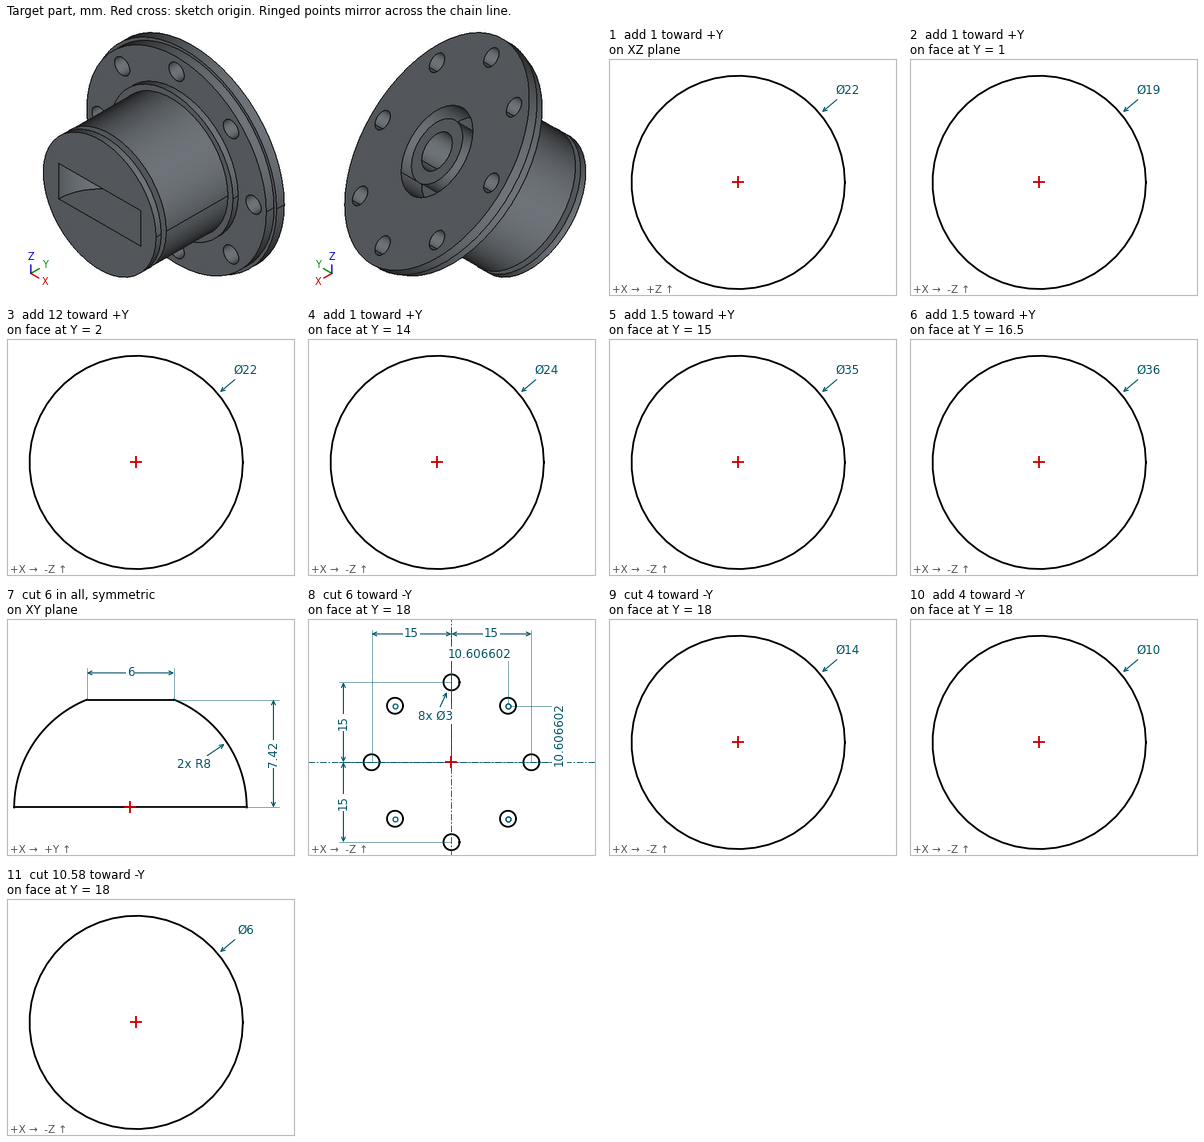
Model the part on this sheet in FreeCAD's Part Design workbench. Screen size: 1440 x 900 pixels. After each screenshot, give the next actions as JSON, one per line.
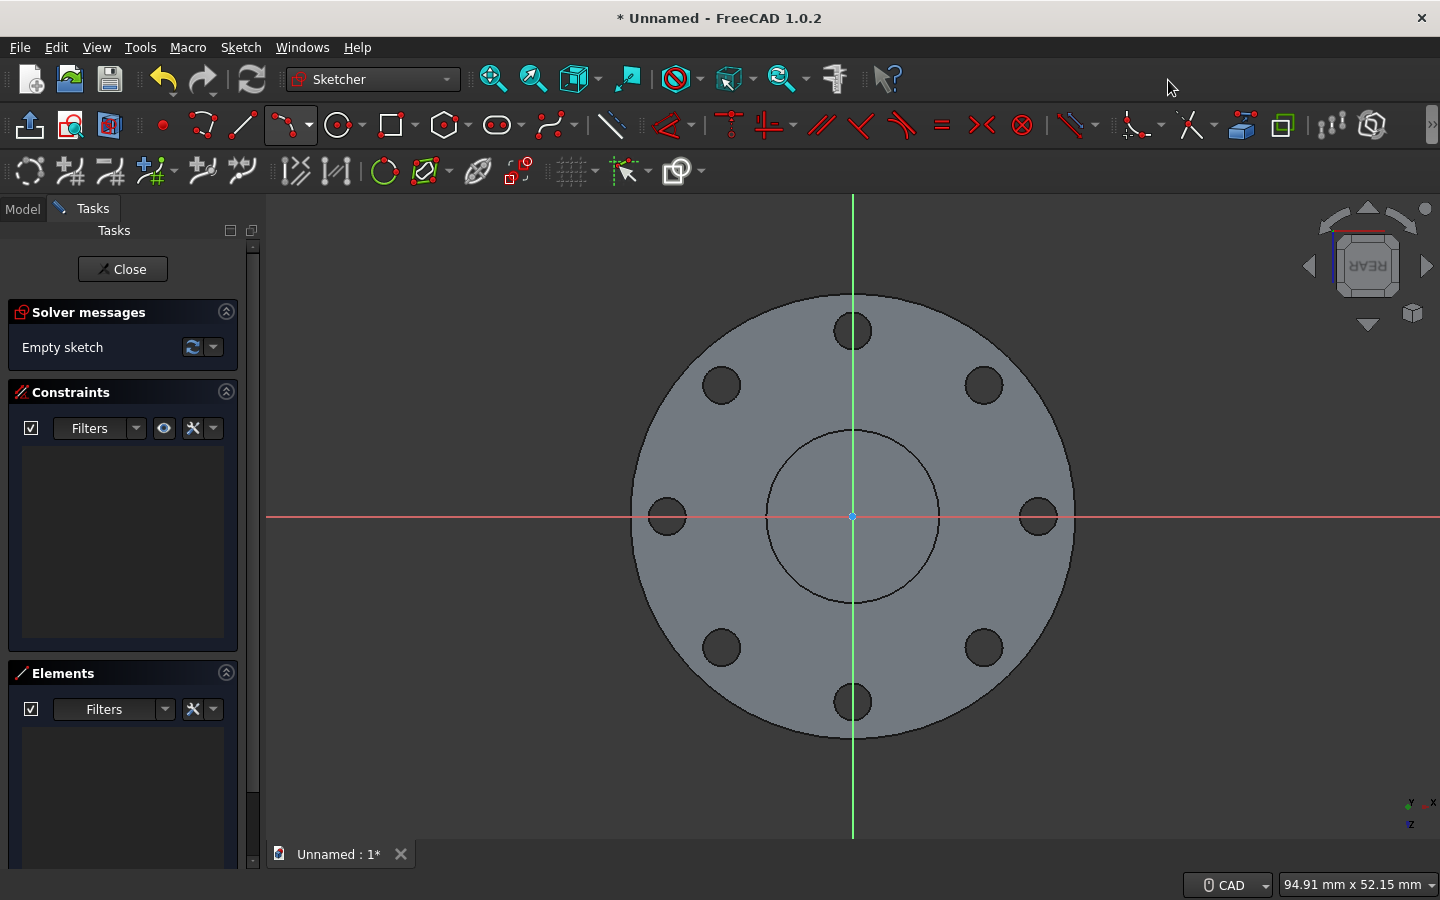
{"action": "scroll", "coordinate": [882, 516], "scroll_direction": "up", "scroll_amount": 6}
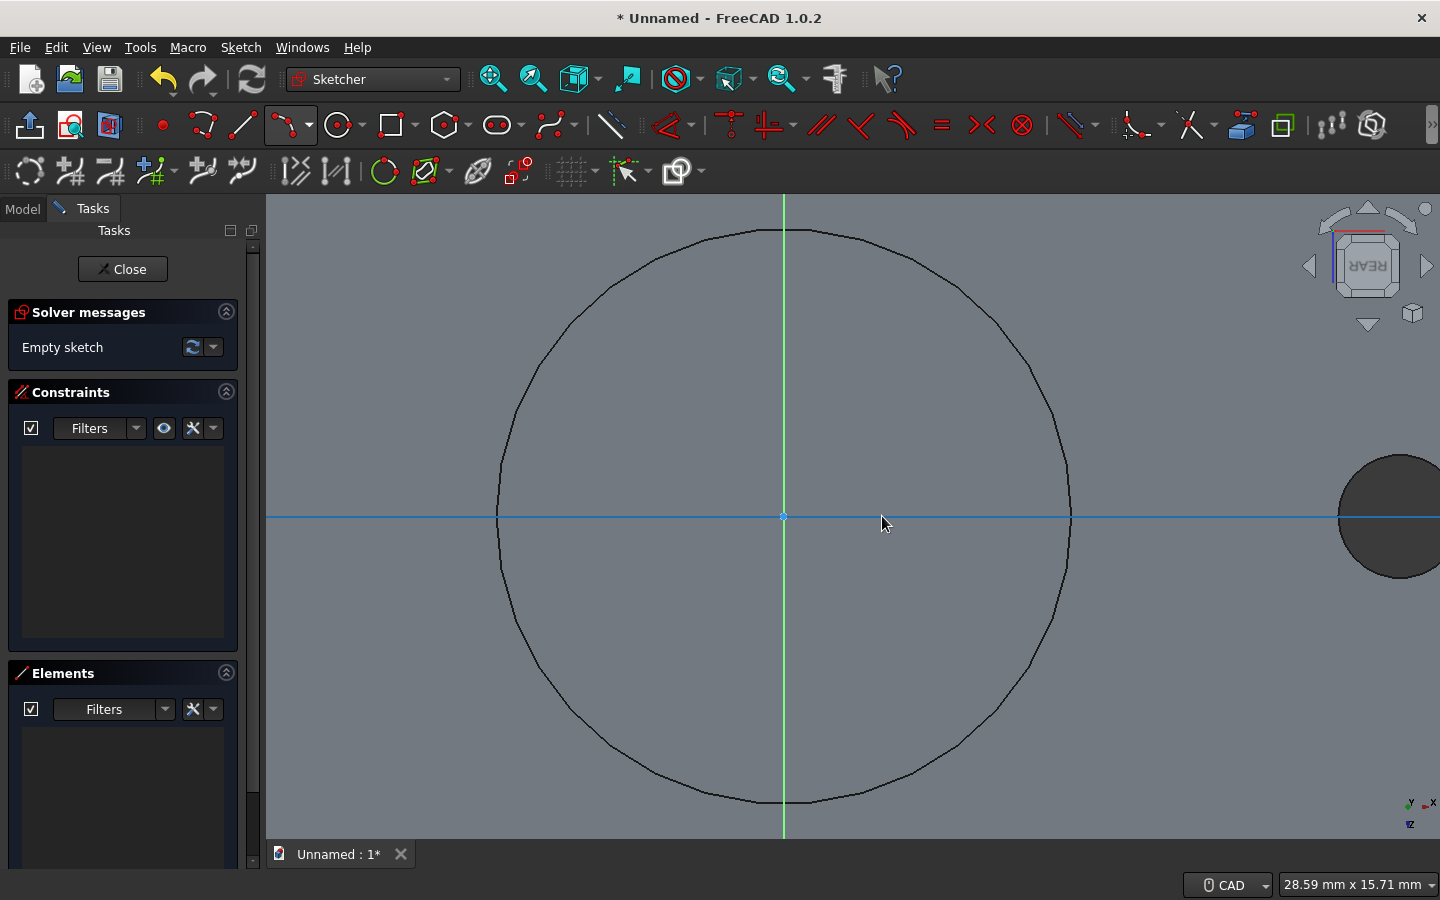
{"action": "left_click", "coordinate": [338, 126]}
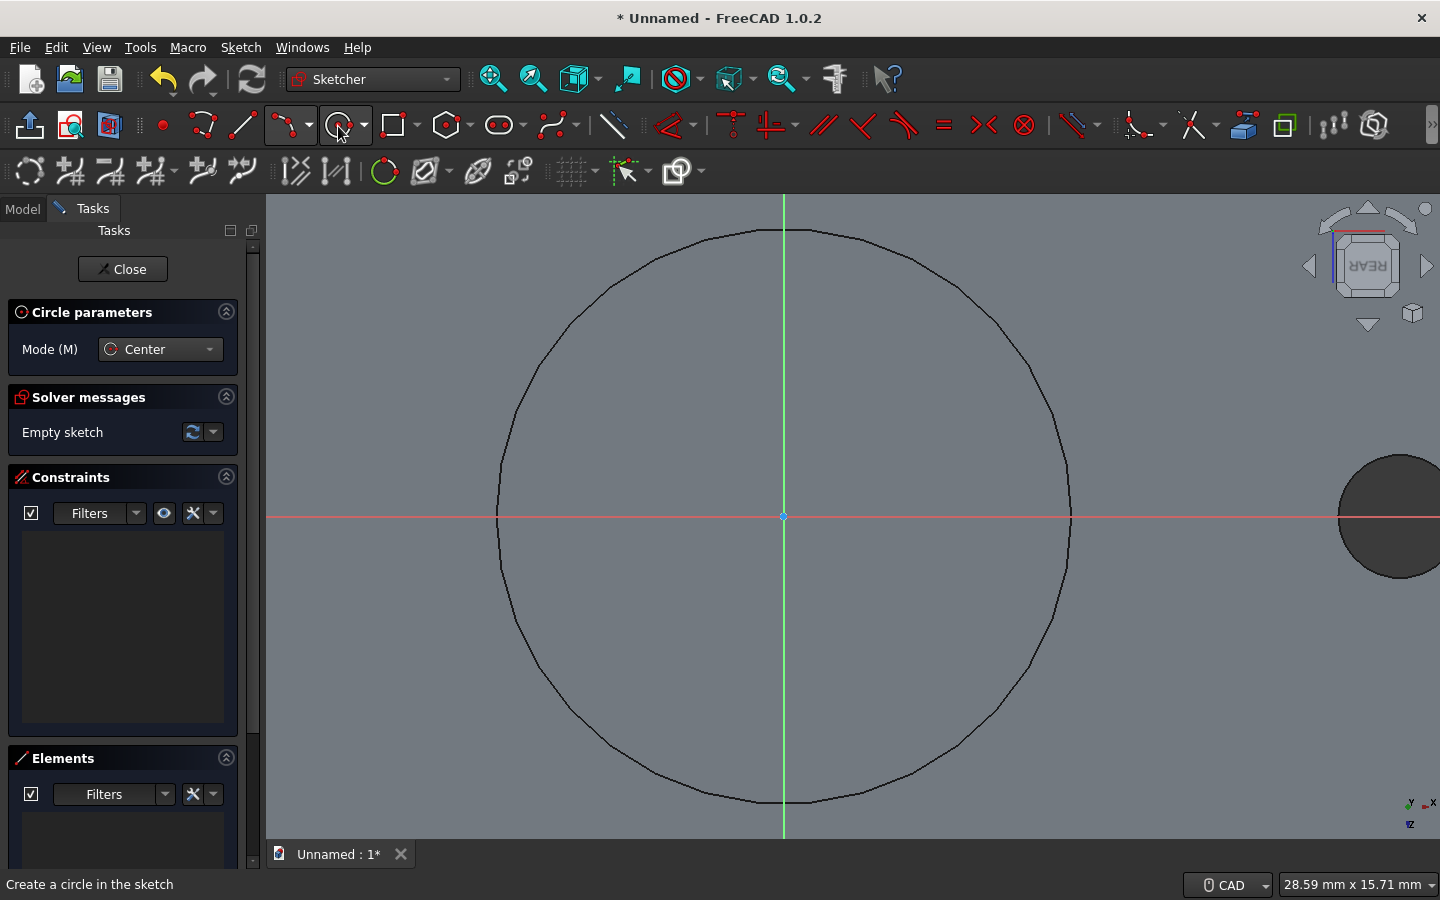
{"action": "left_click", "coordinate": [784, 516]}
{"action": "mouse_move", "coordinate": [929, 371]}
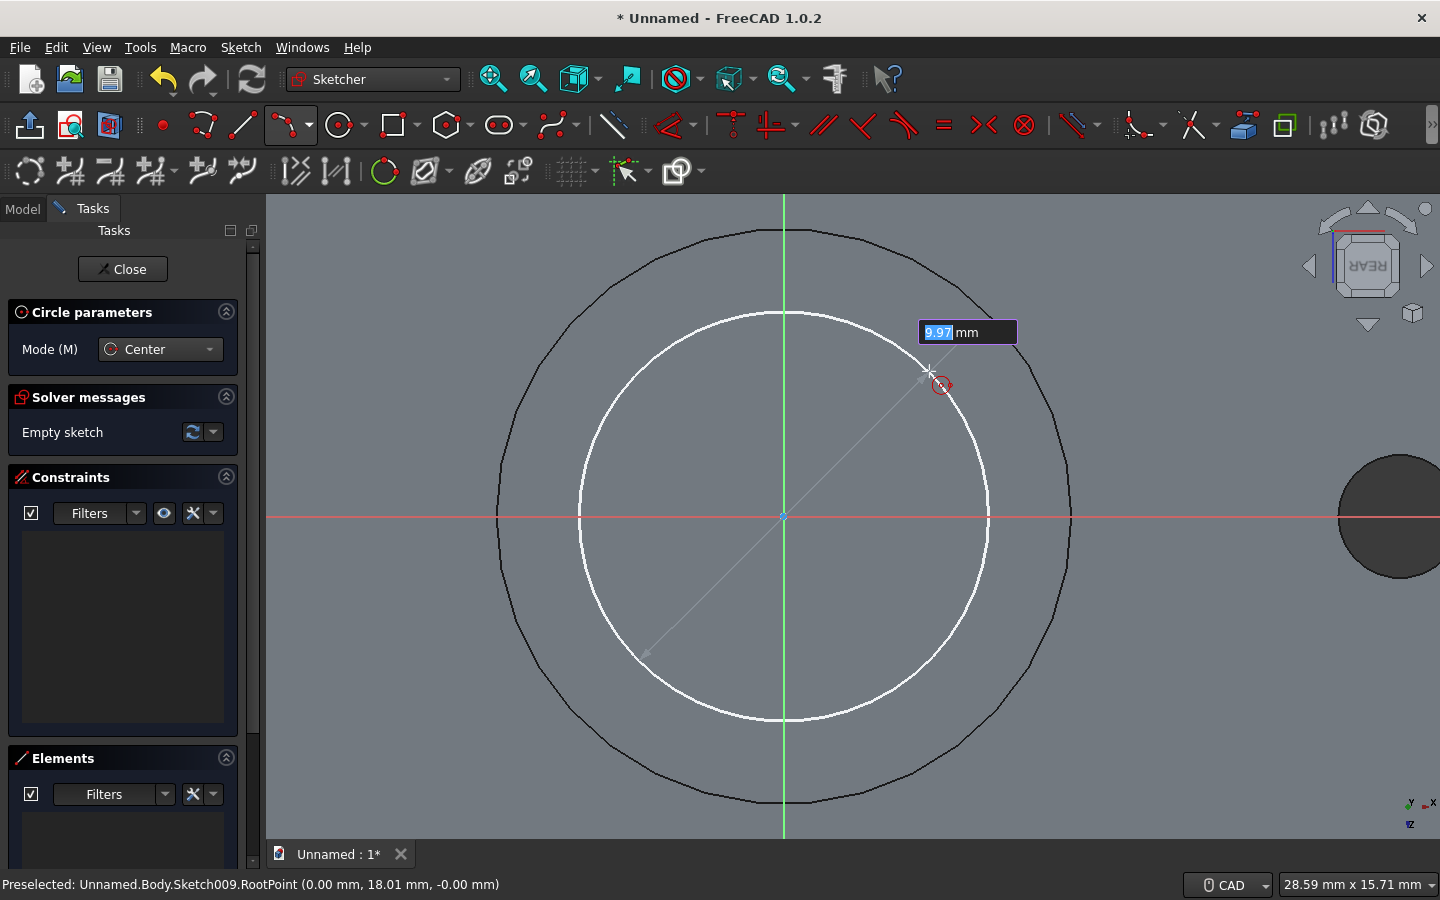
{"action": "type", "text": "10"}
{"action": "key", "text": "Return"}
{"action": "key", "text": "Escape"}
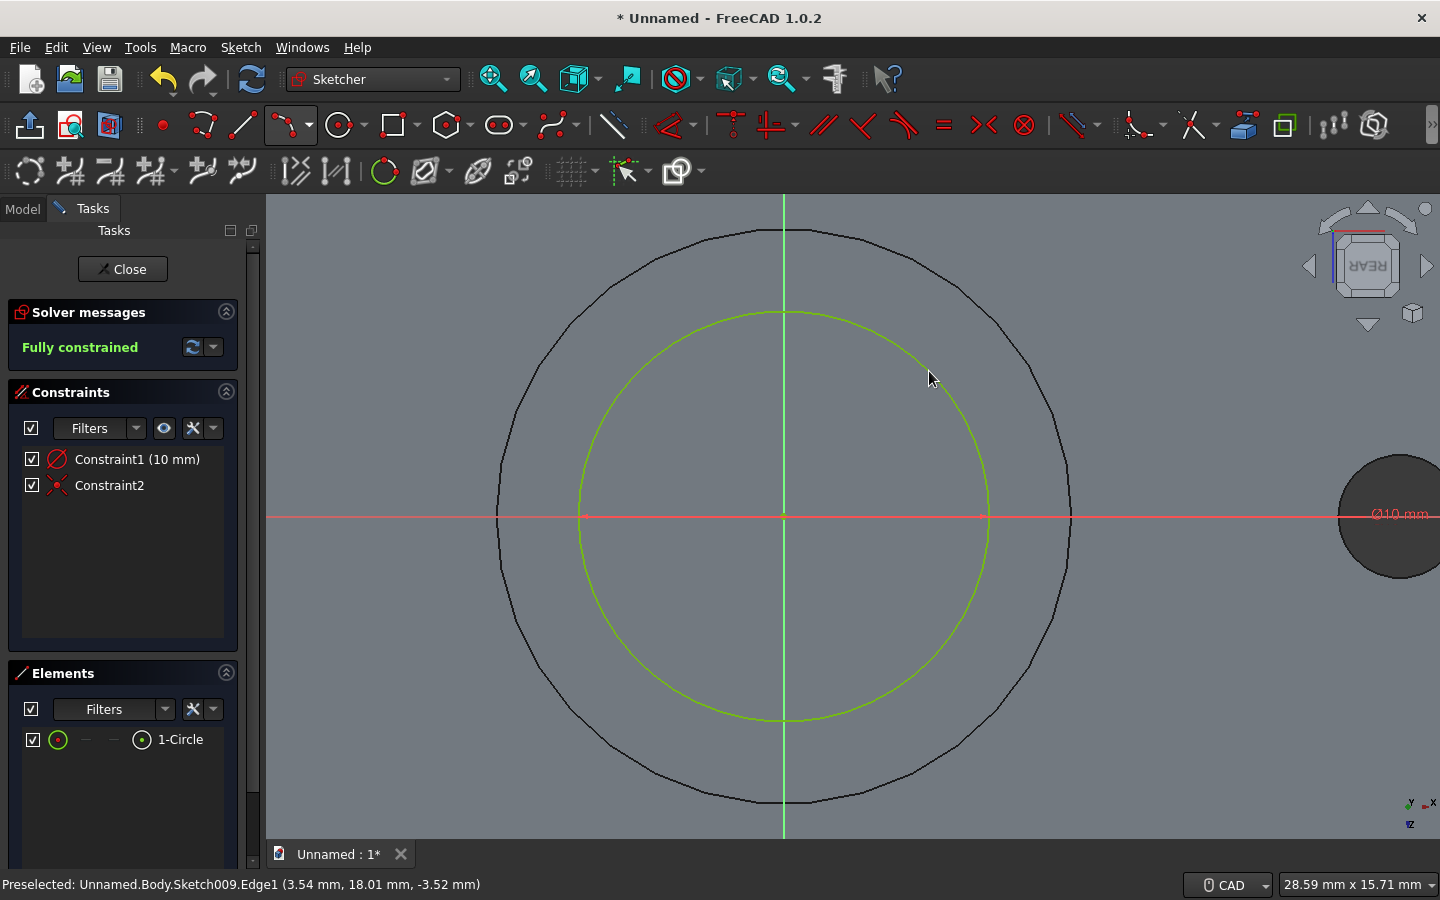
{"action": "left_click", "coordinate": [123, 269]}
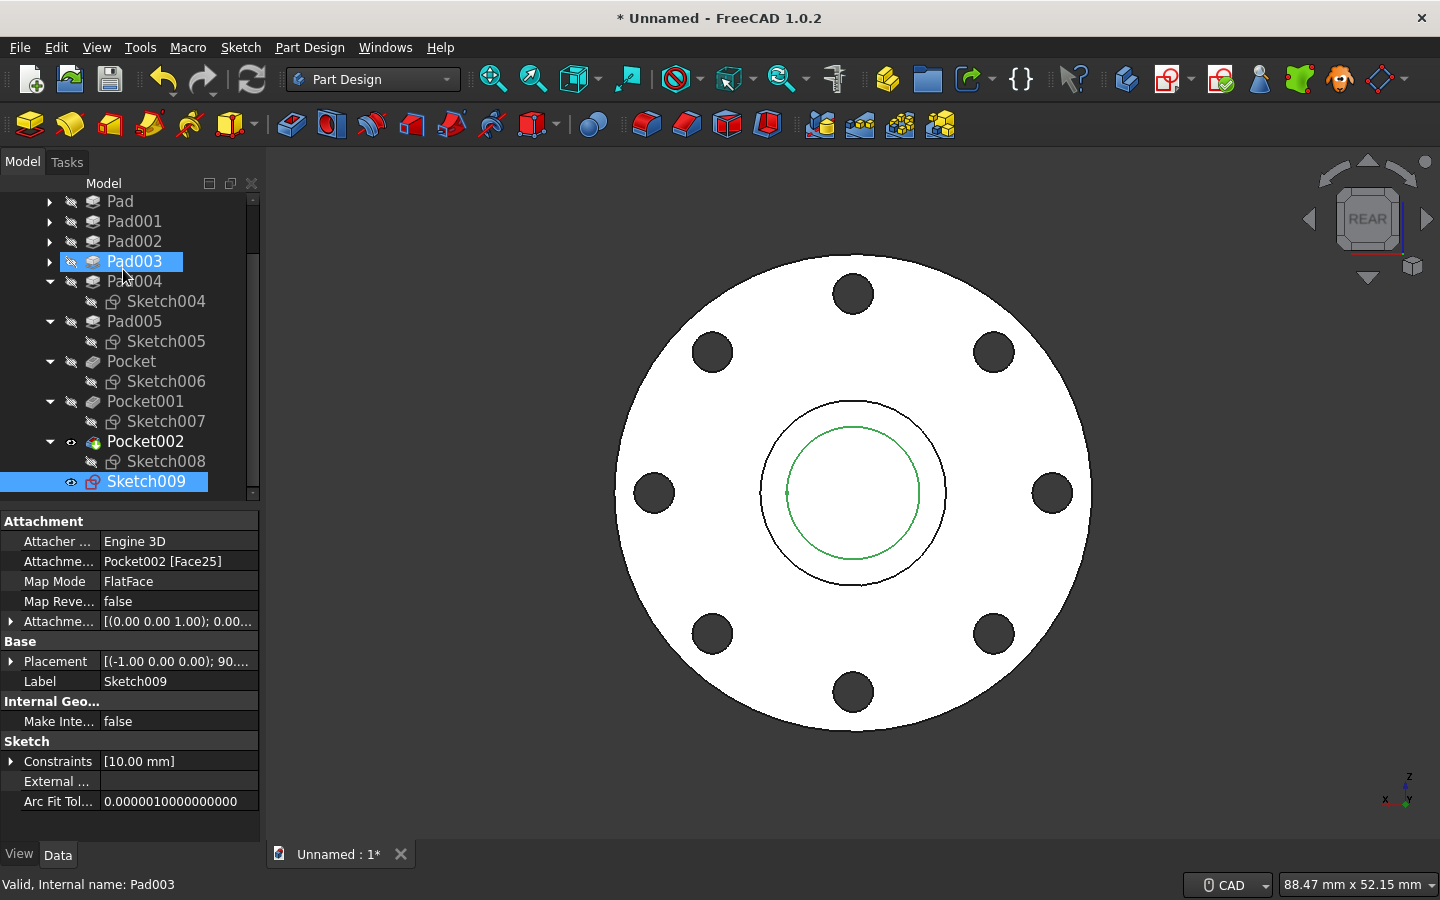
{"action": "left_click", "coordinate": [30, 124]}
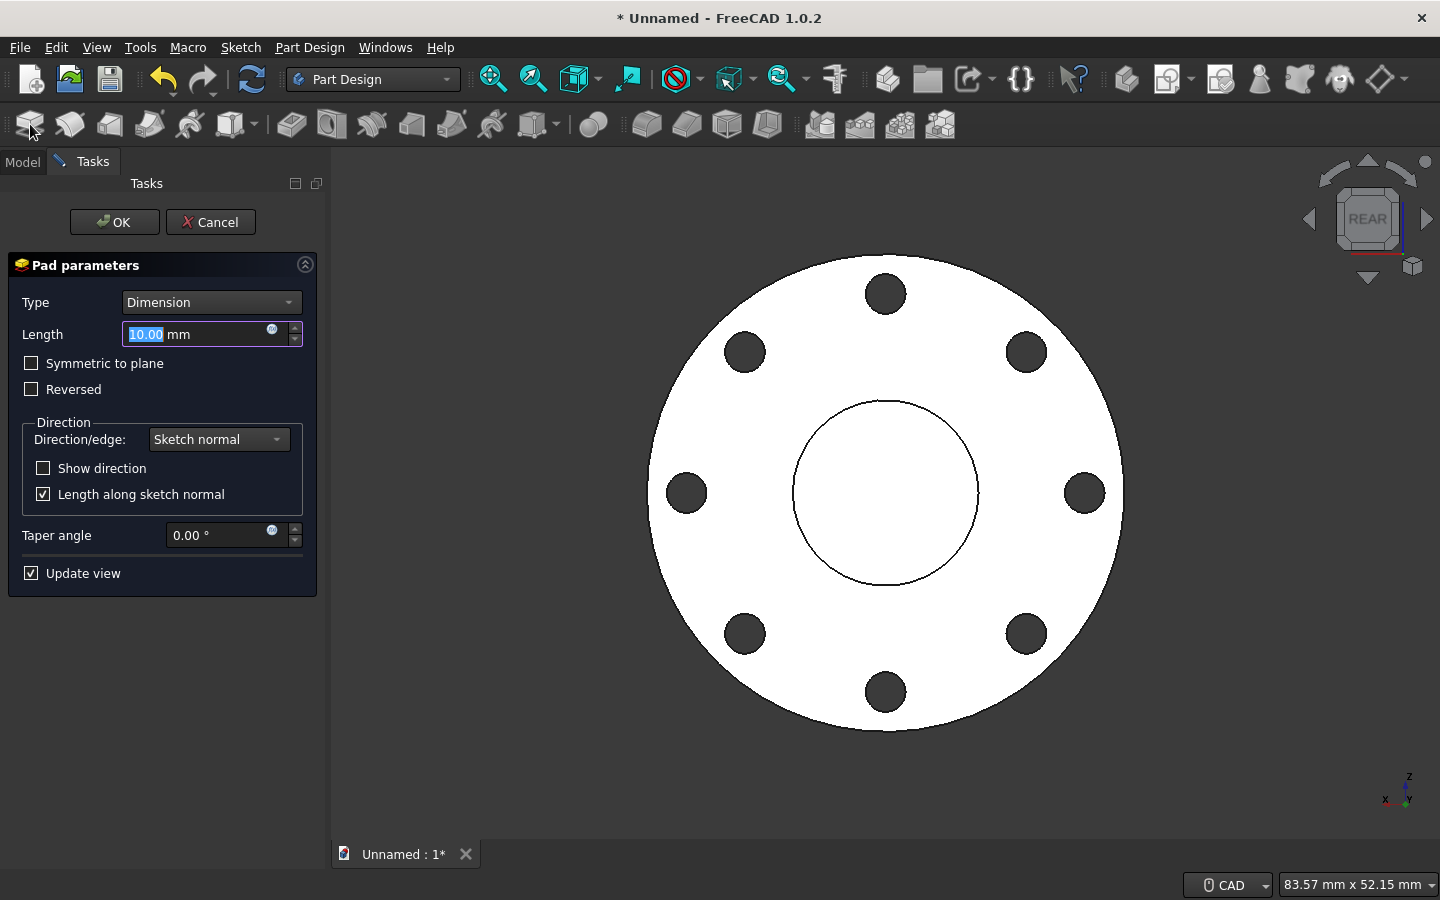
{"action": "type", "text": "4"}
{"action": "key", "text": "Tab"}